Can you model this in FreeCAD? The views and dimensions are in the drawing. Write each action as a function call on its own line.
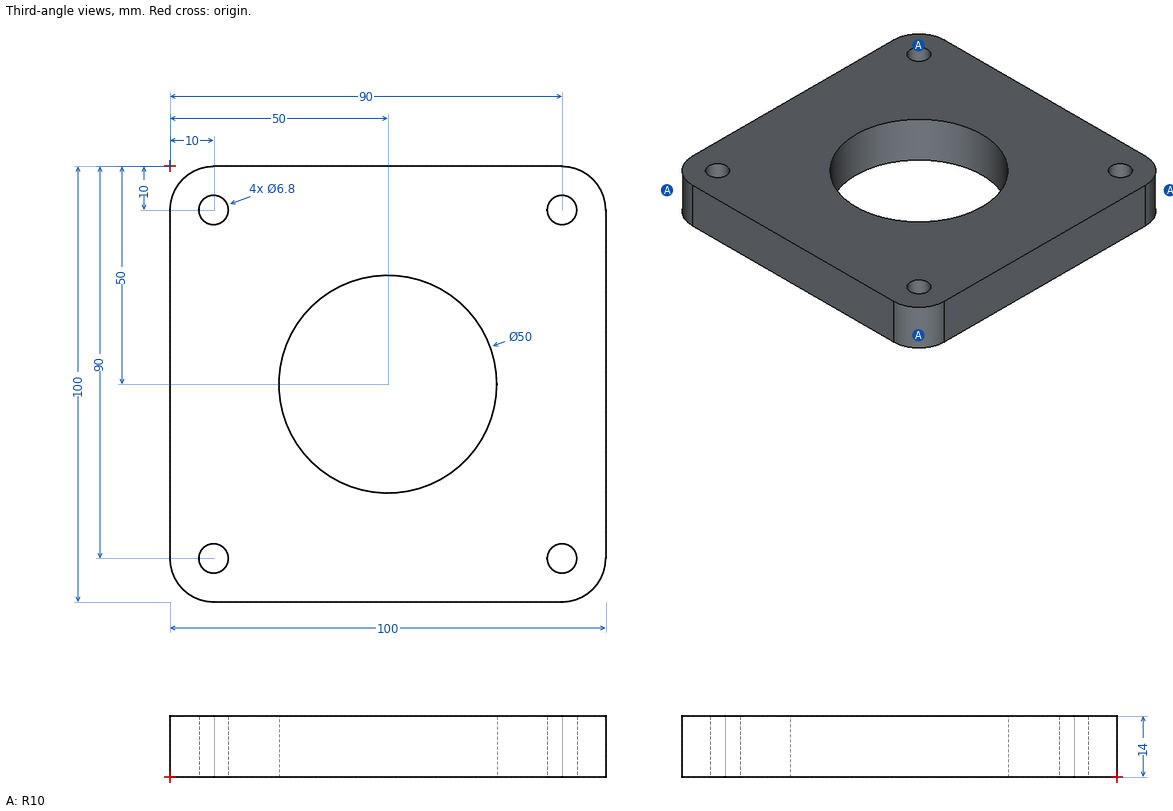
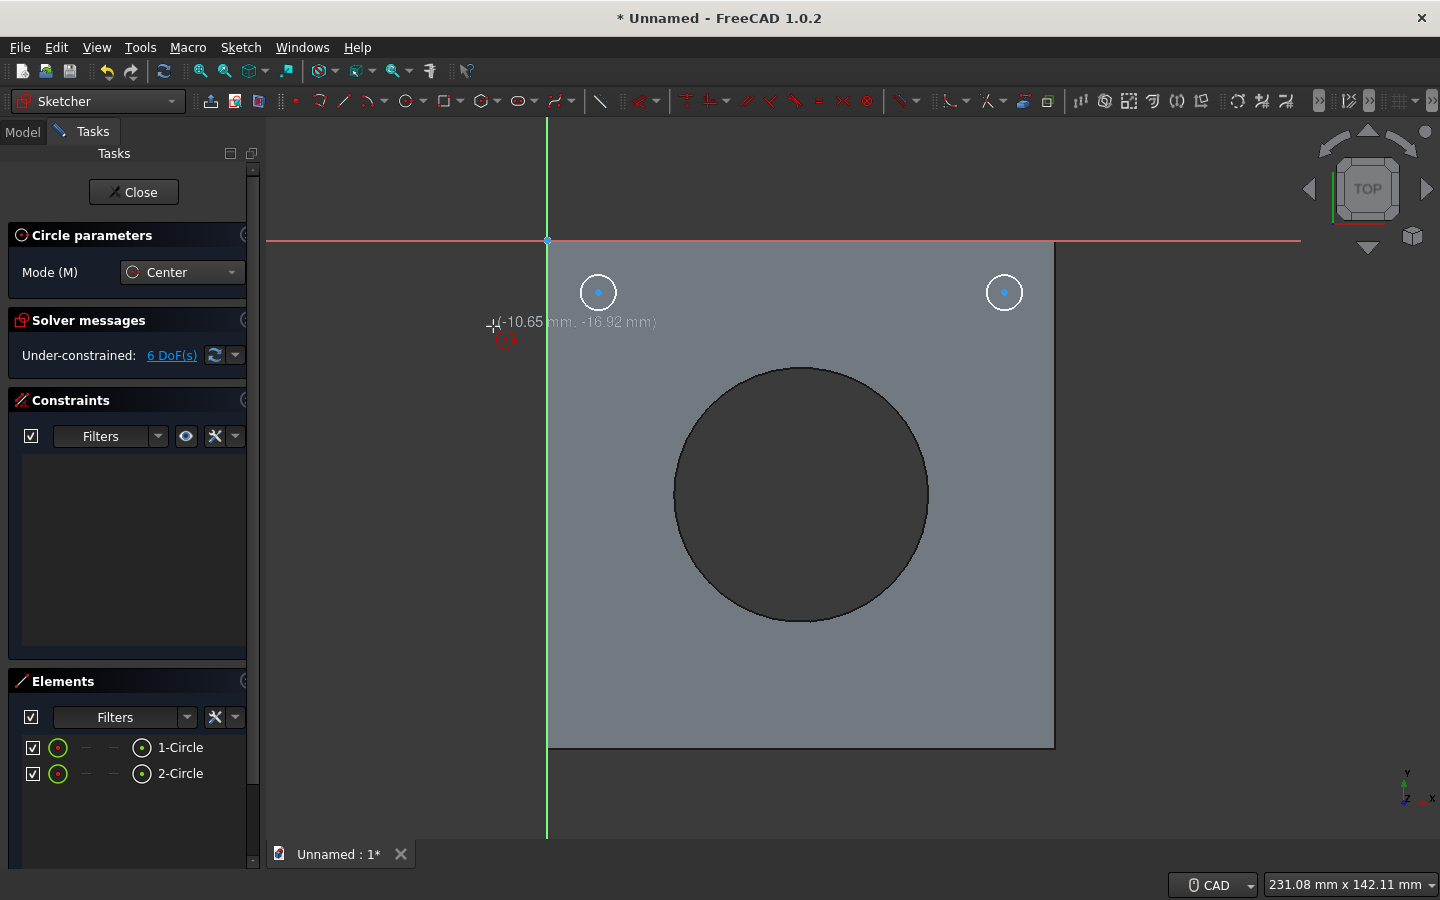
scroll(598, 698, up, 2)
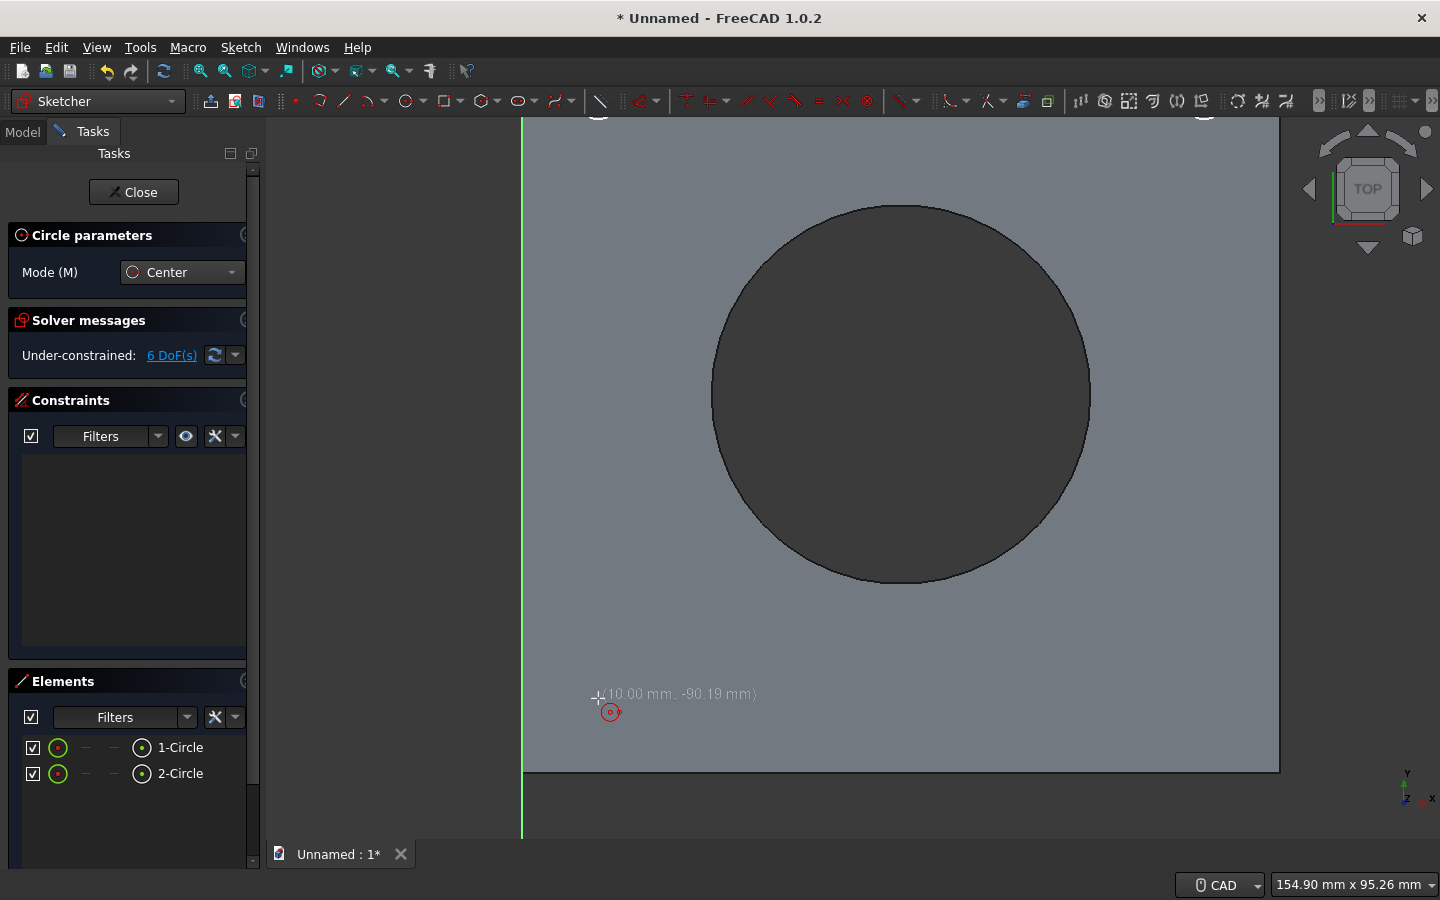
click(598, 698)
click(616, 679)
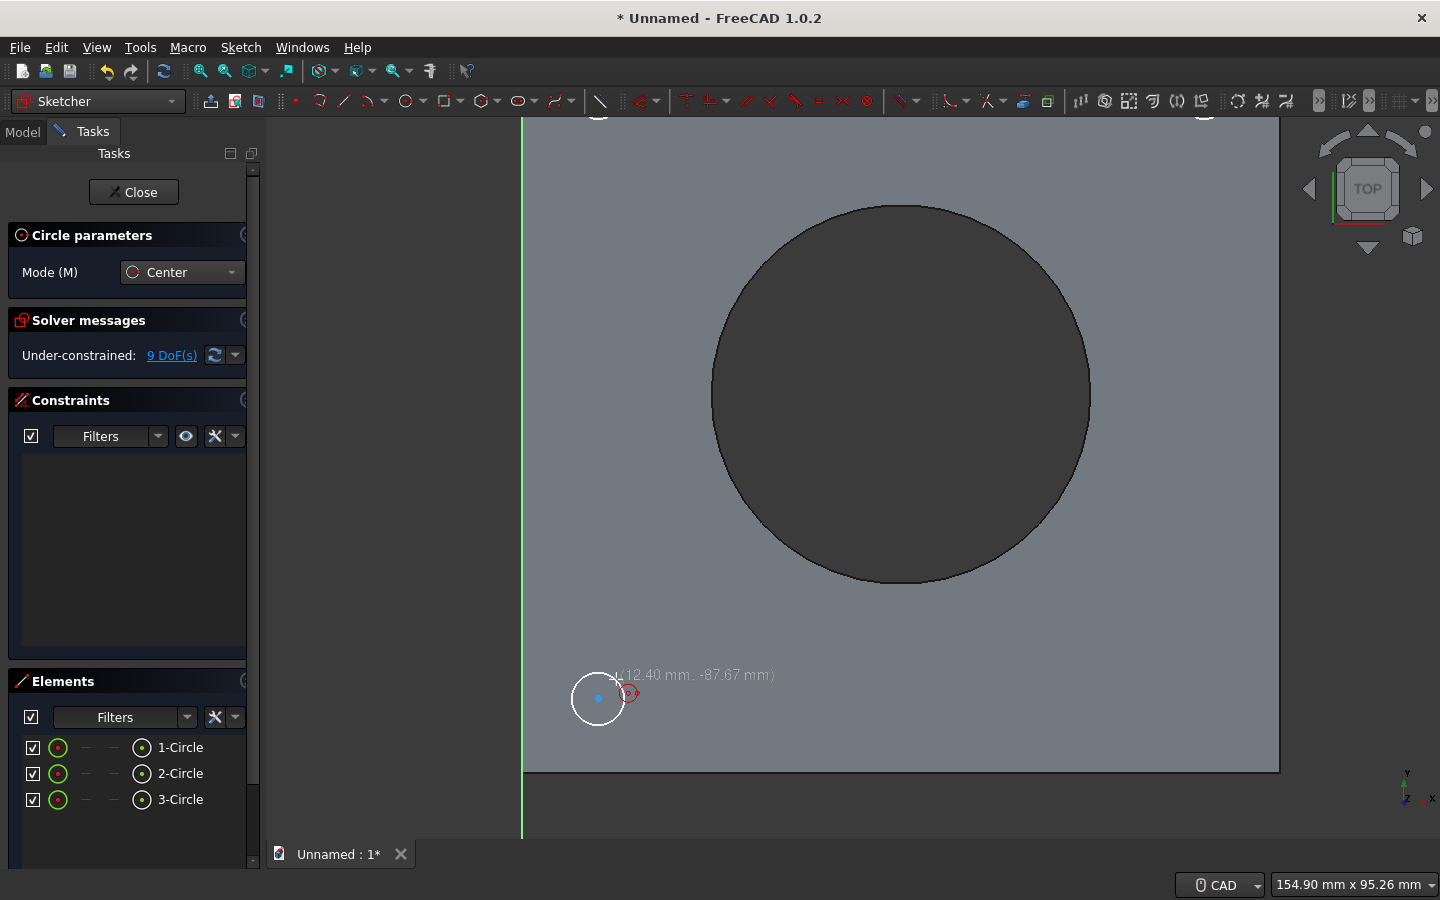
click(1204, 698)
click(1222, 679)
key(Escape)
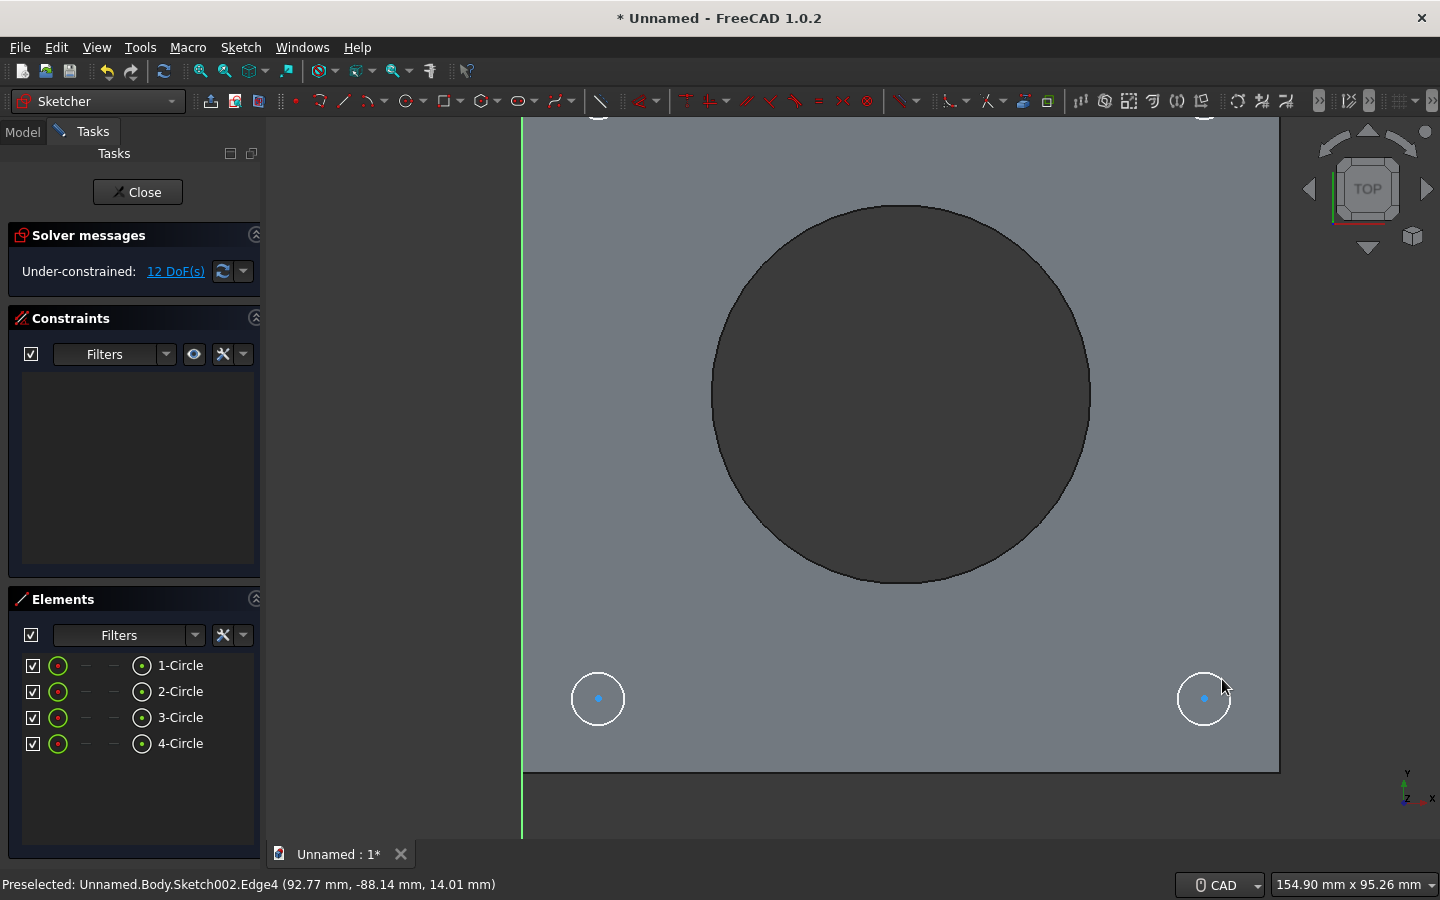
scroll(598, 699, down, 2)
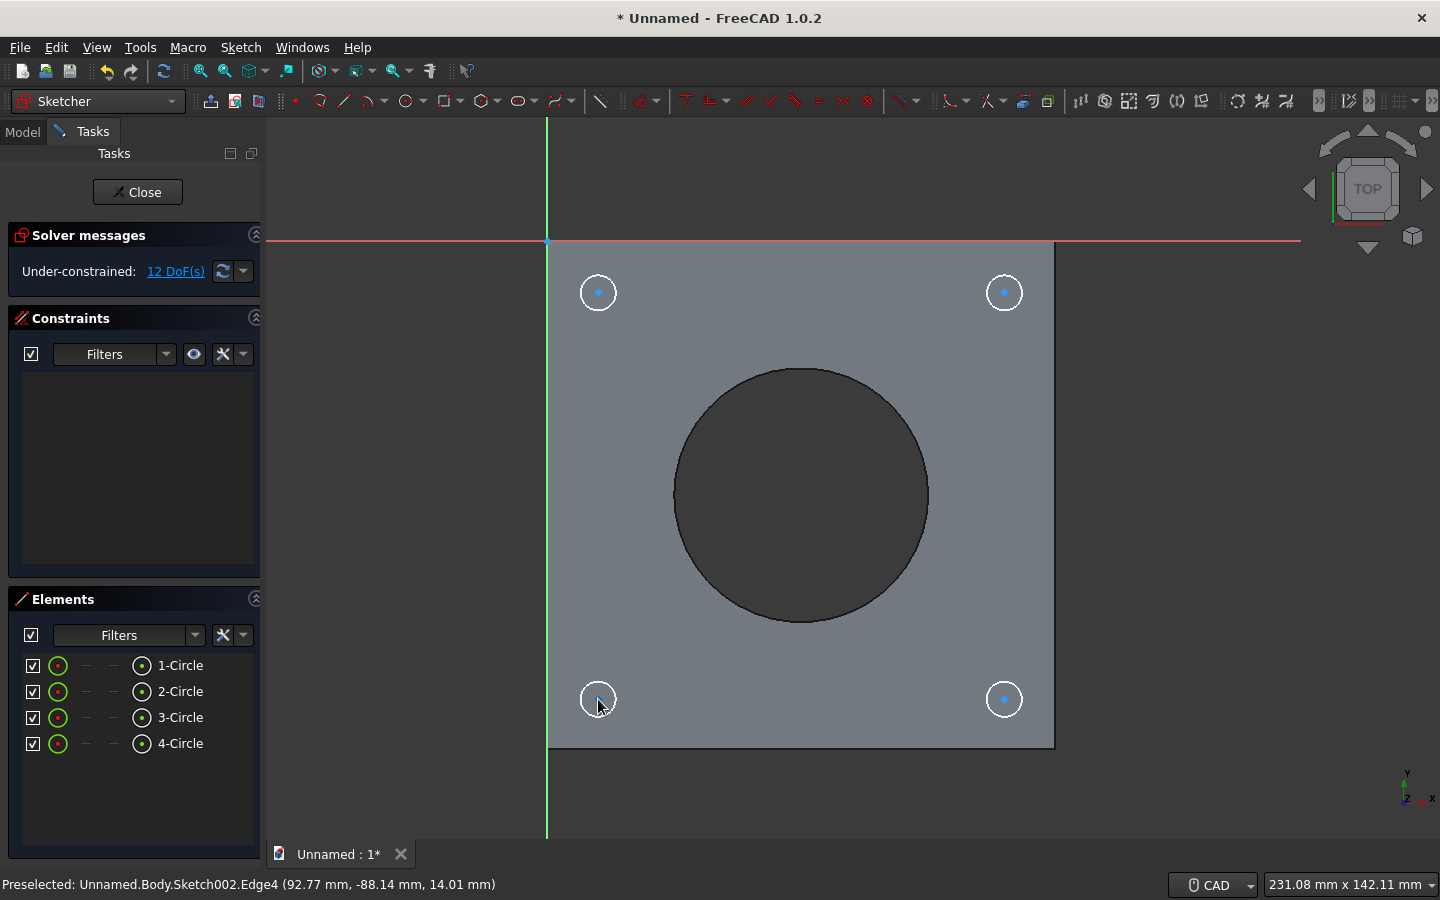
click(611, 280)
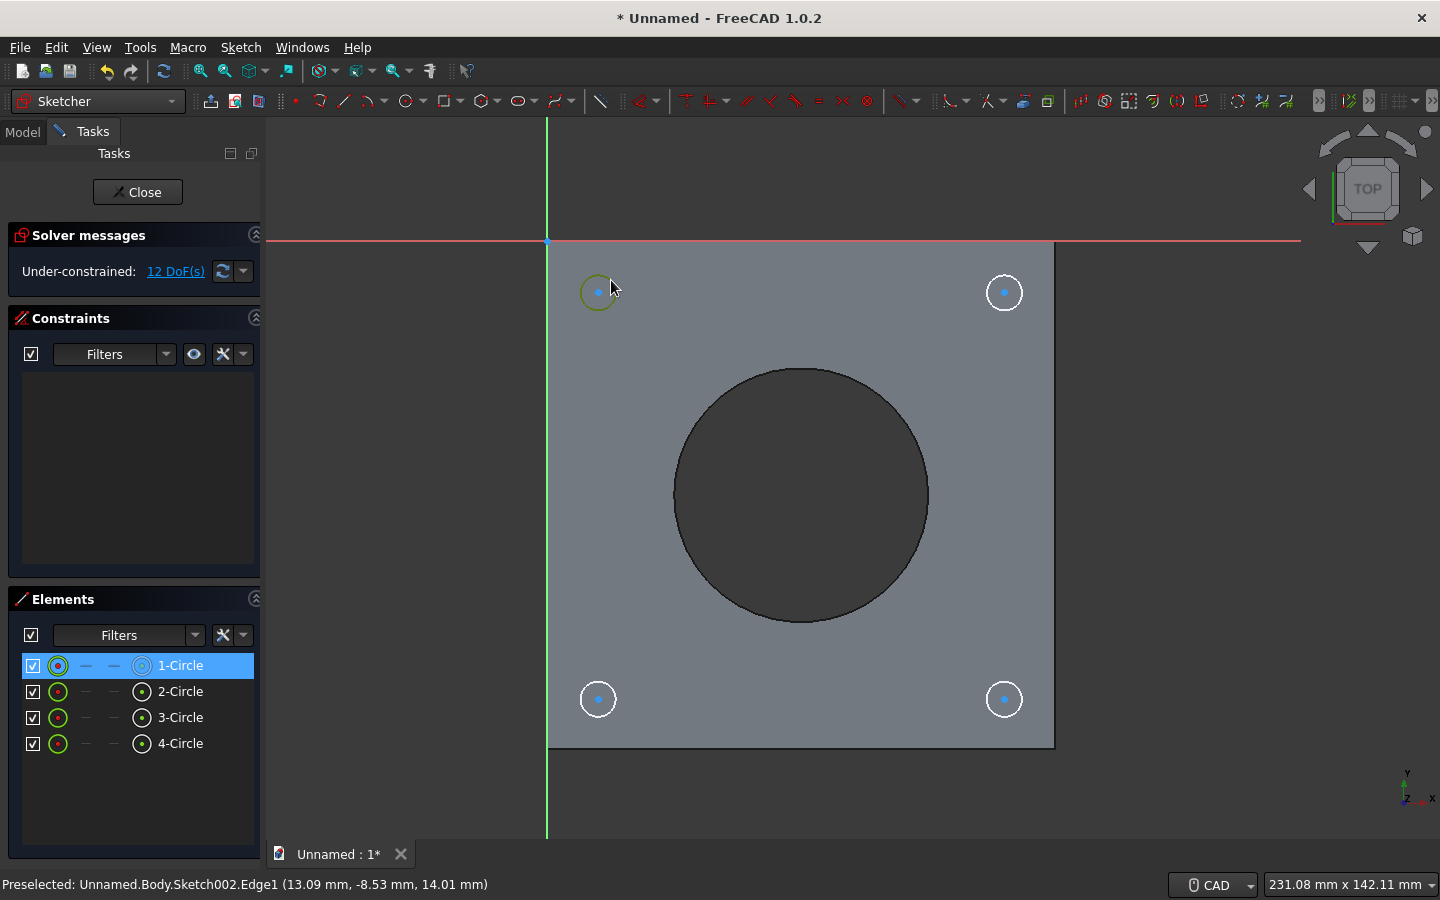
click(1017, 280)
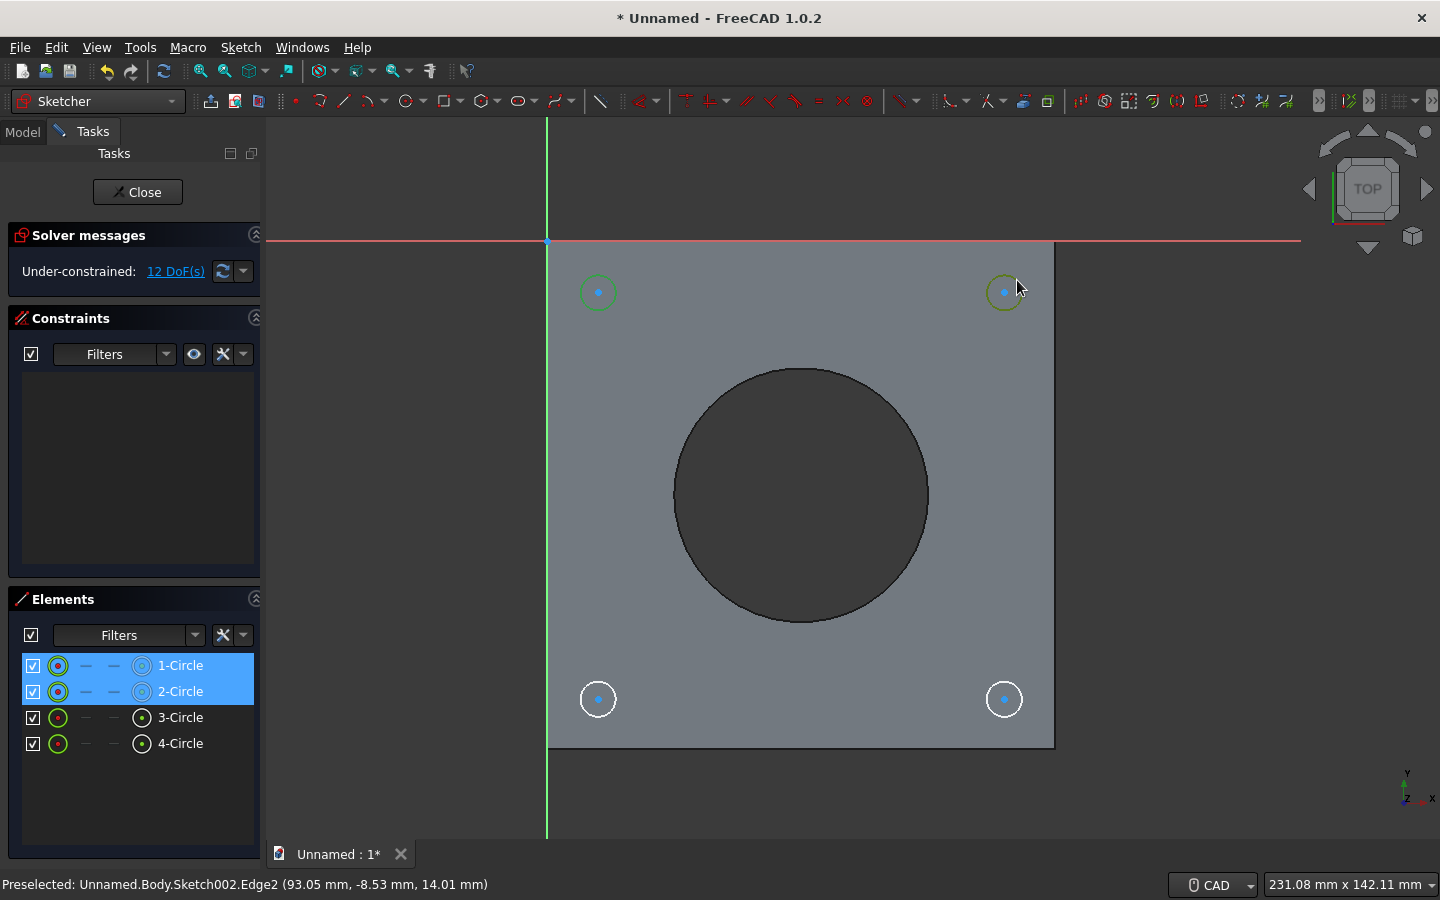
click(610, 687)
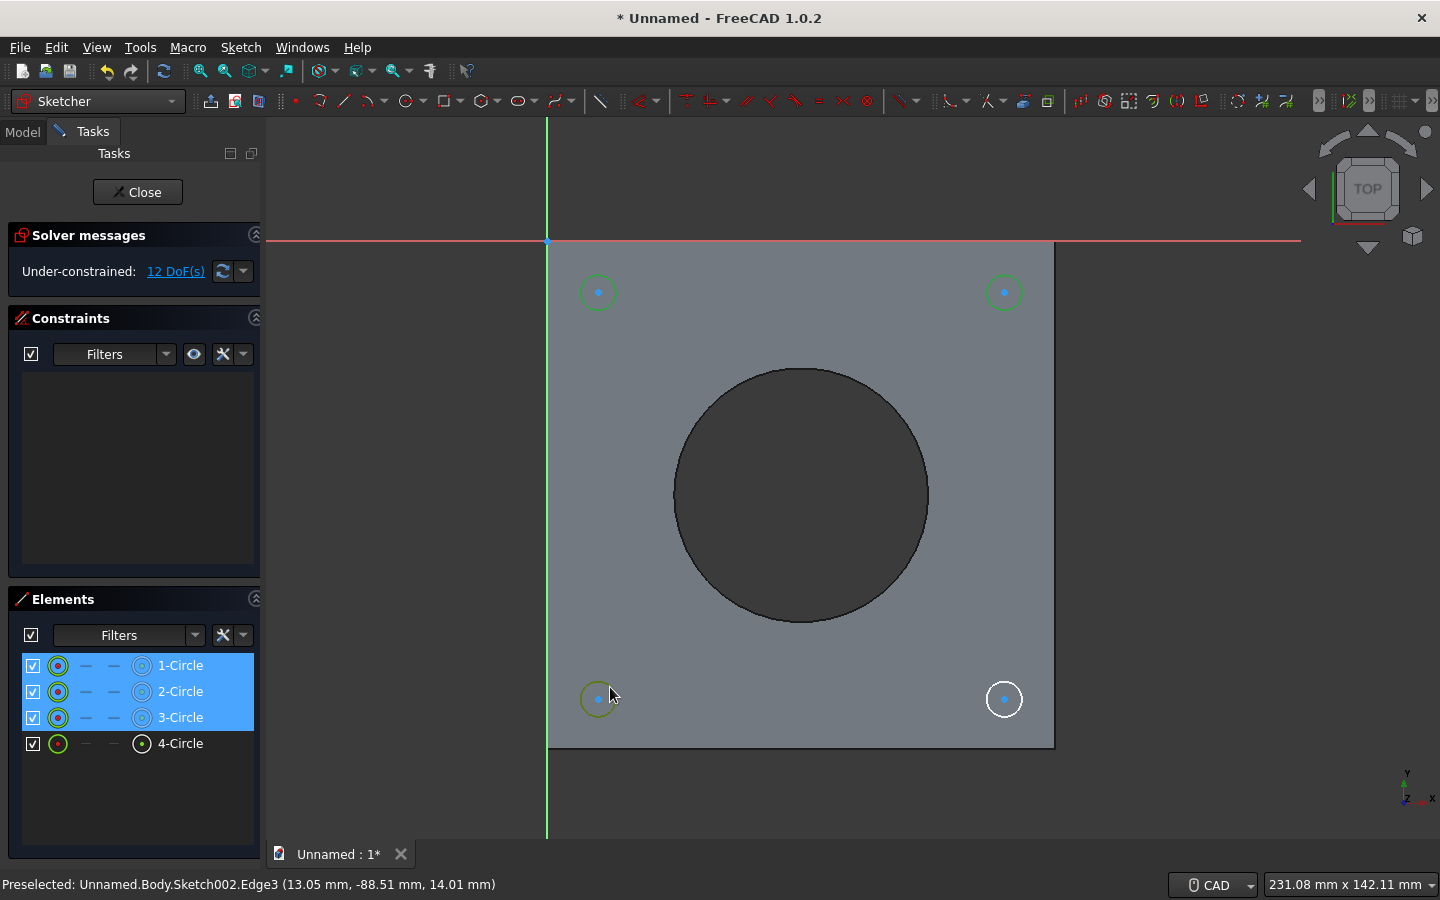
click(1017, 687)